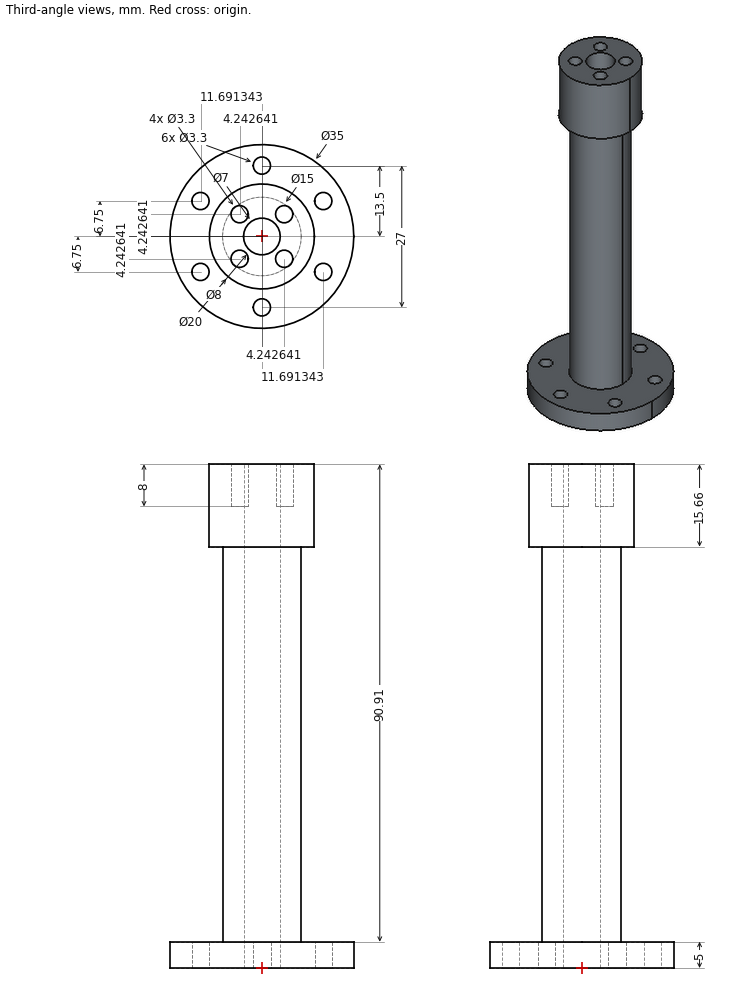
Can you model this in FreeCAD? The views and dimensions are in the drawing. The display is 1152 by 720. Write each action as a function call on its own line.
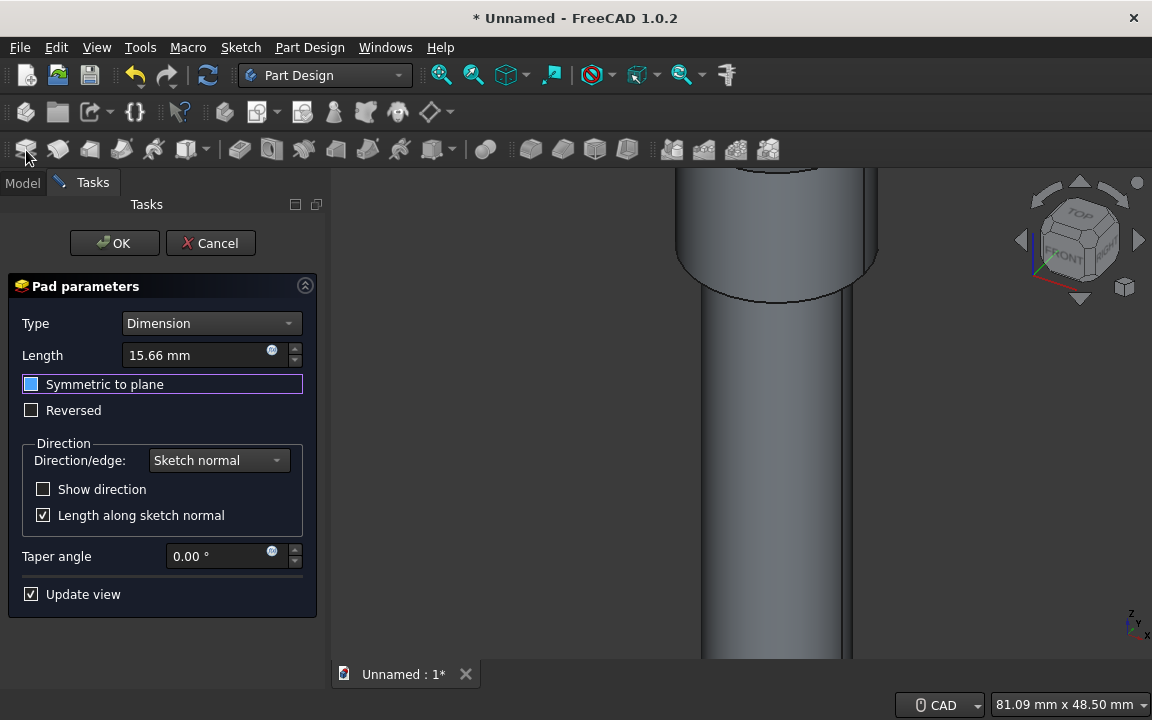
click(30, 410)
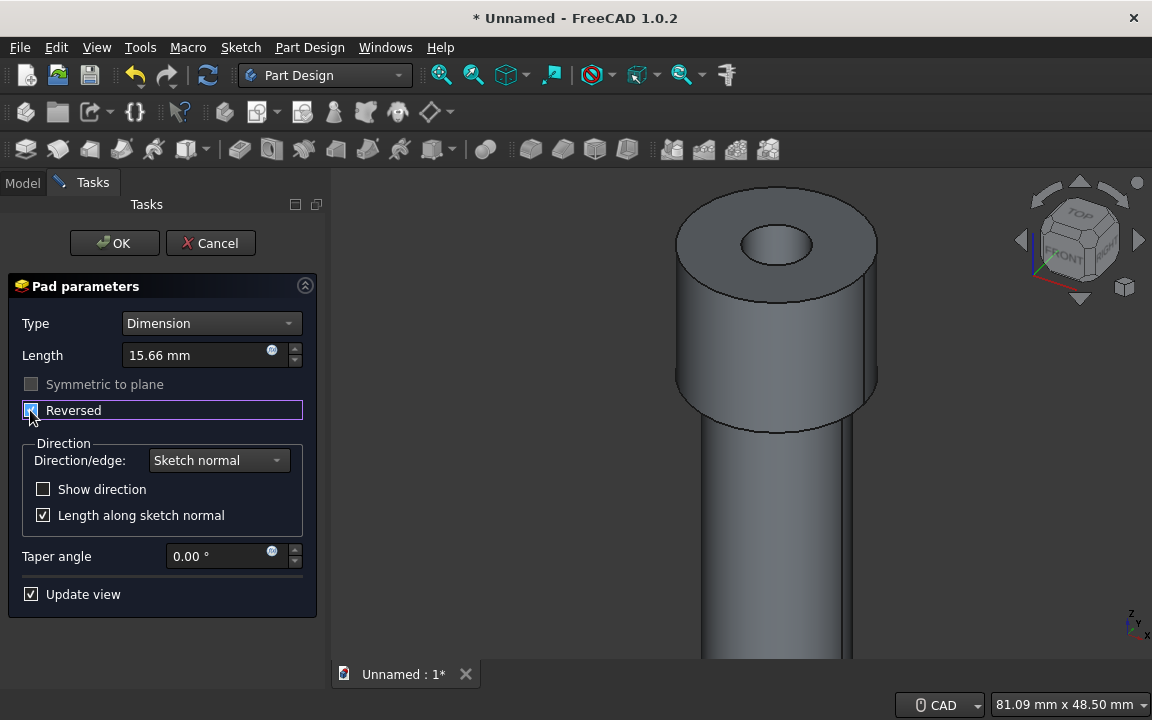
click(115, 243)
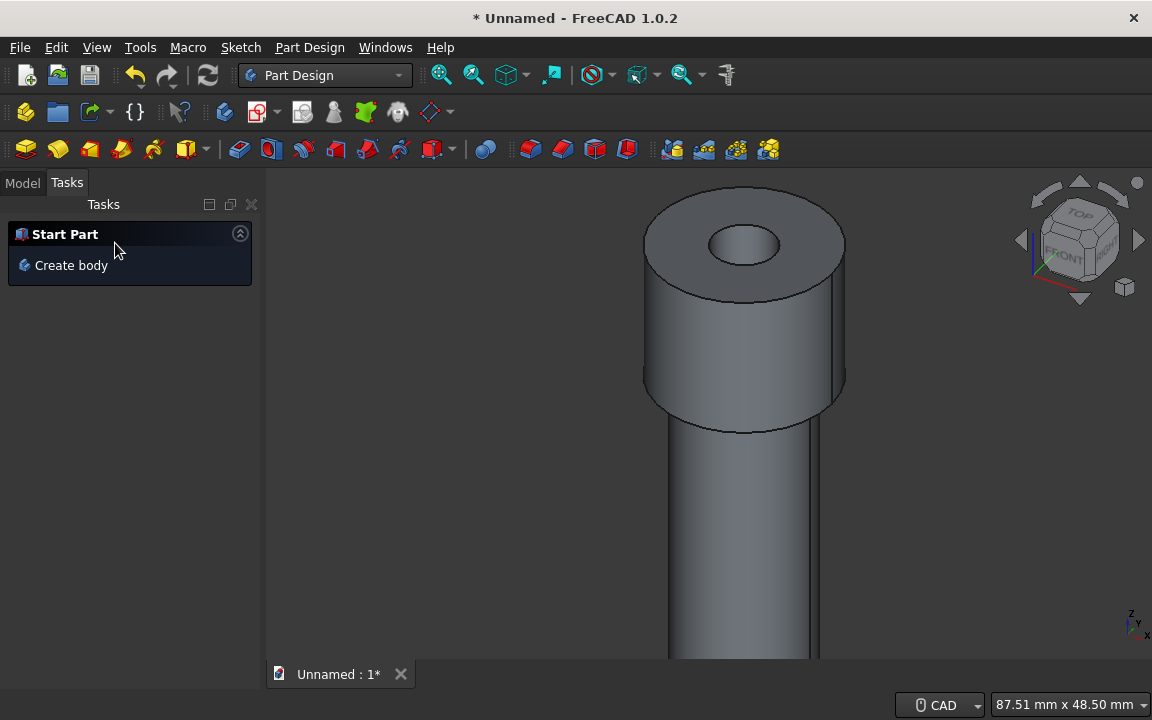
key(v)
key(f)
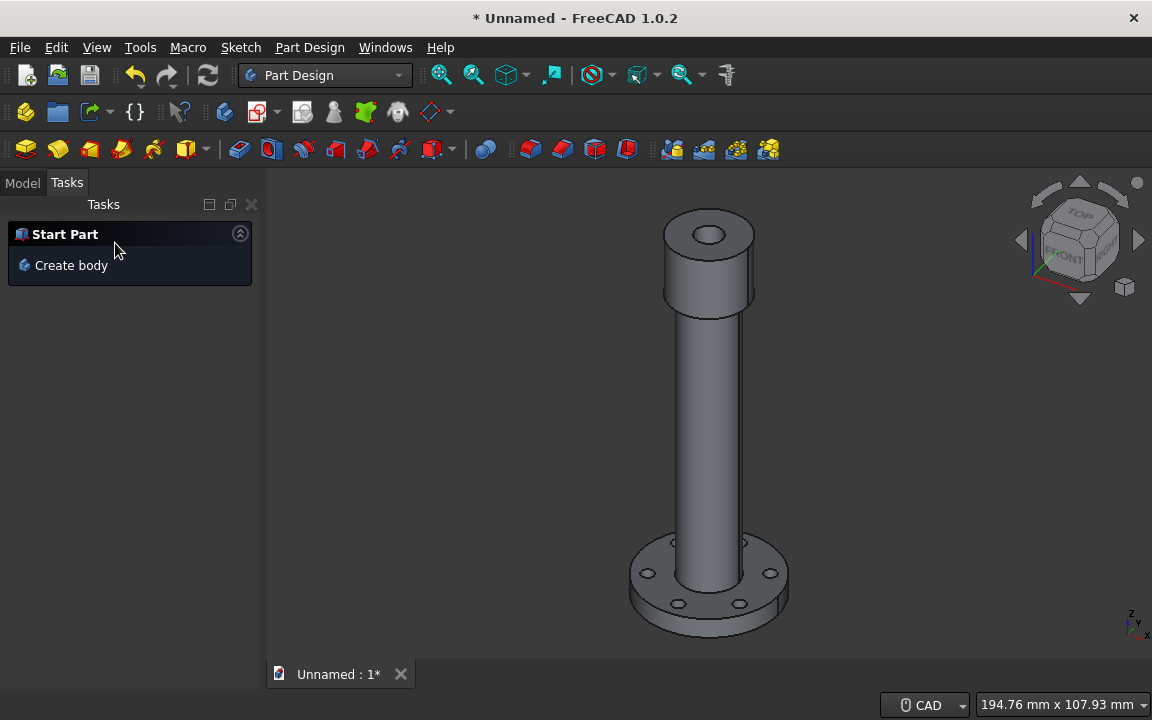
click(680, 233)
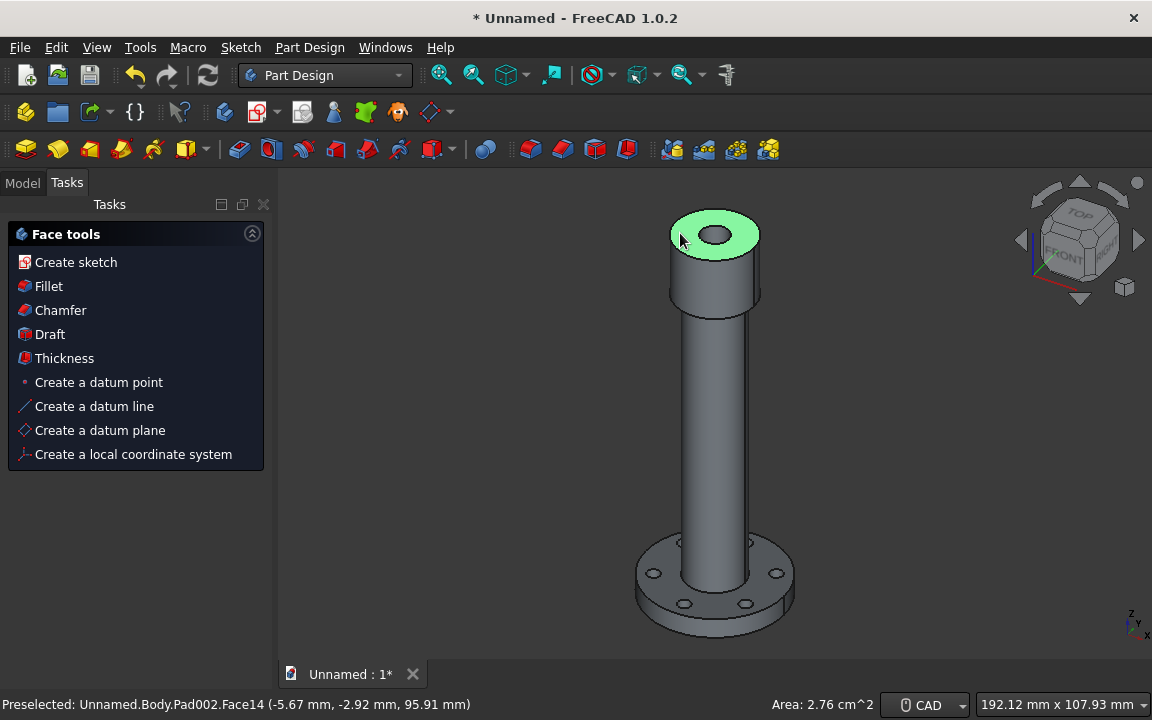
click(258, 112)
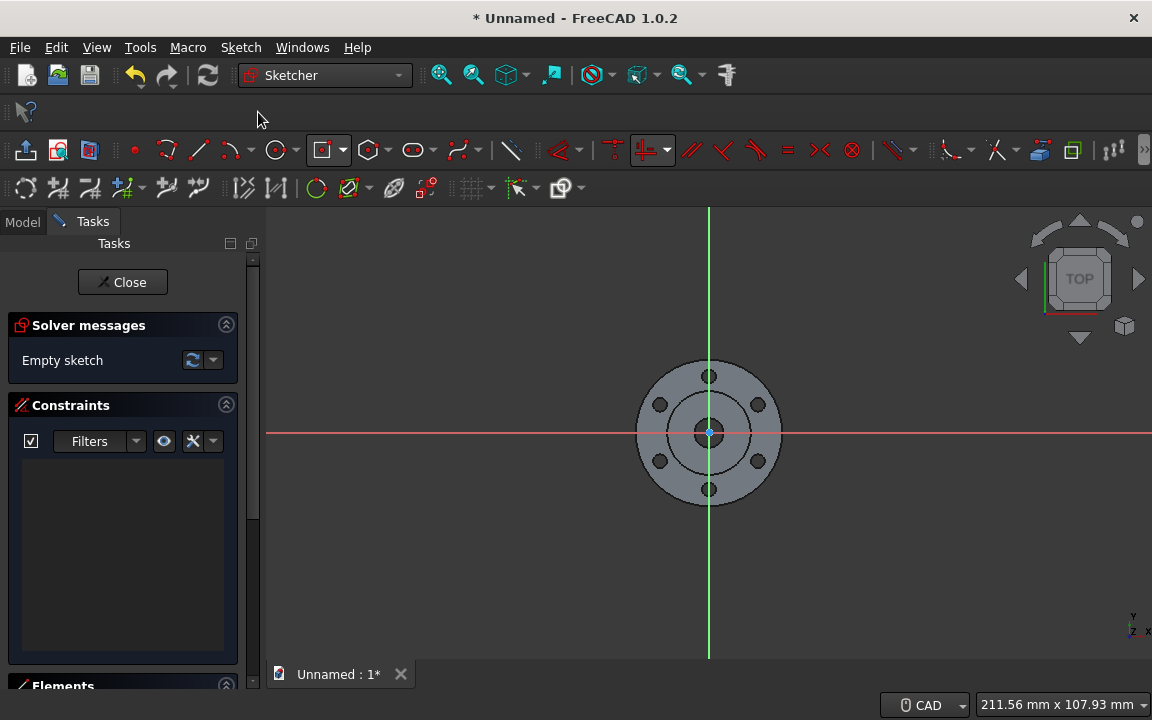
scroll(723, 433, up, 9)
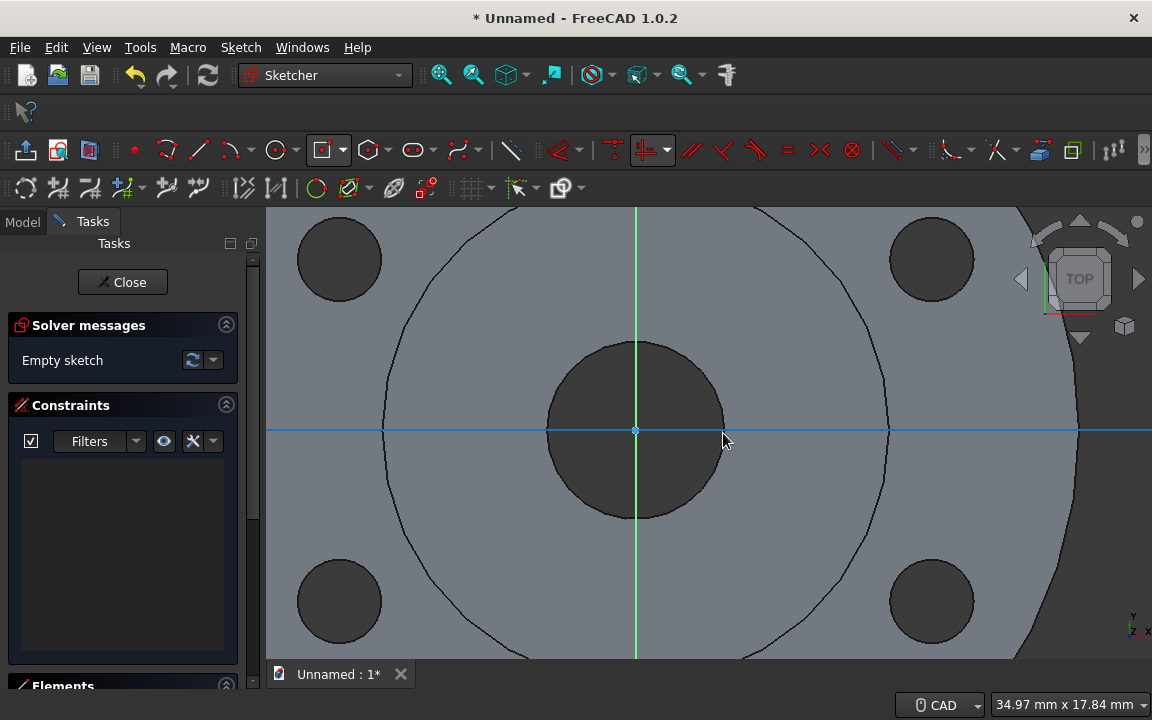
click(276, 150)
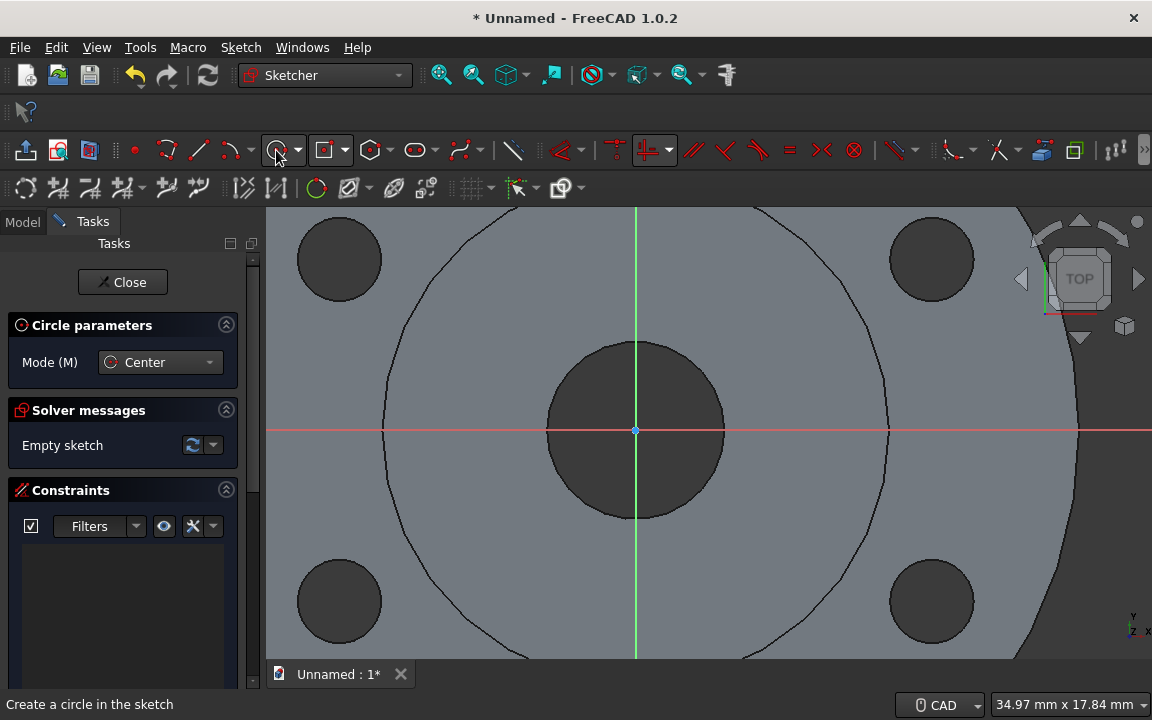
click(528, 323)
click(558, 293)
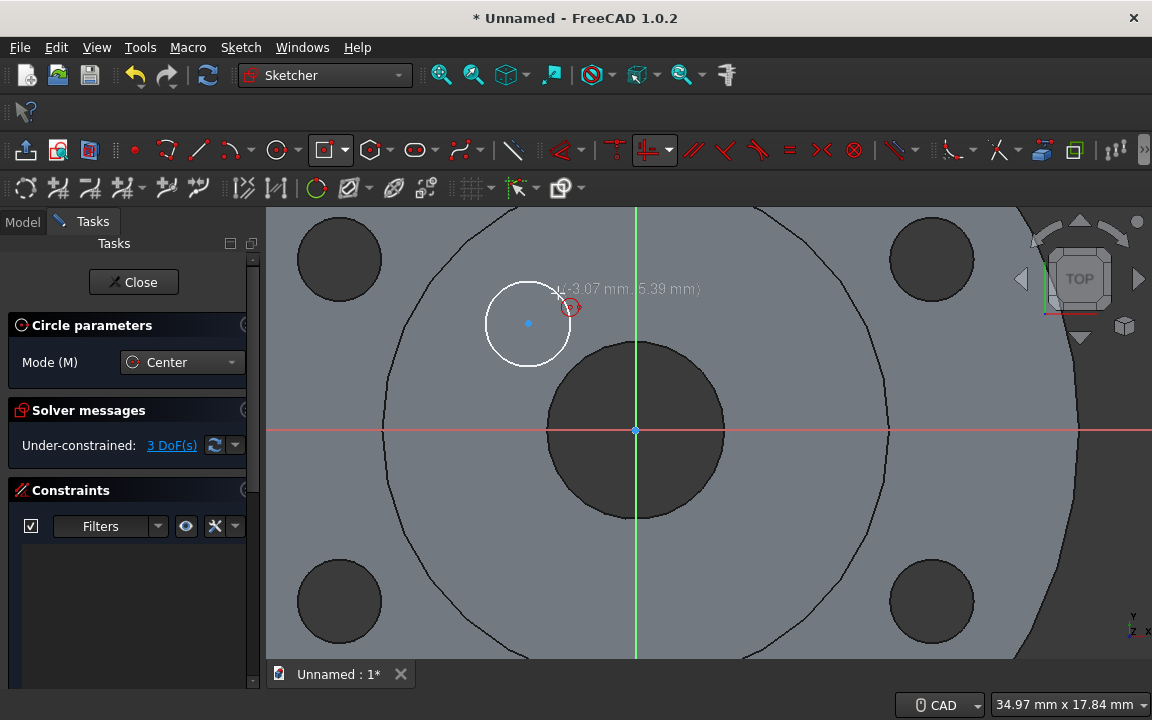
click(528, 538)
click(558, 508)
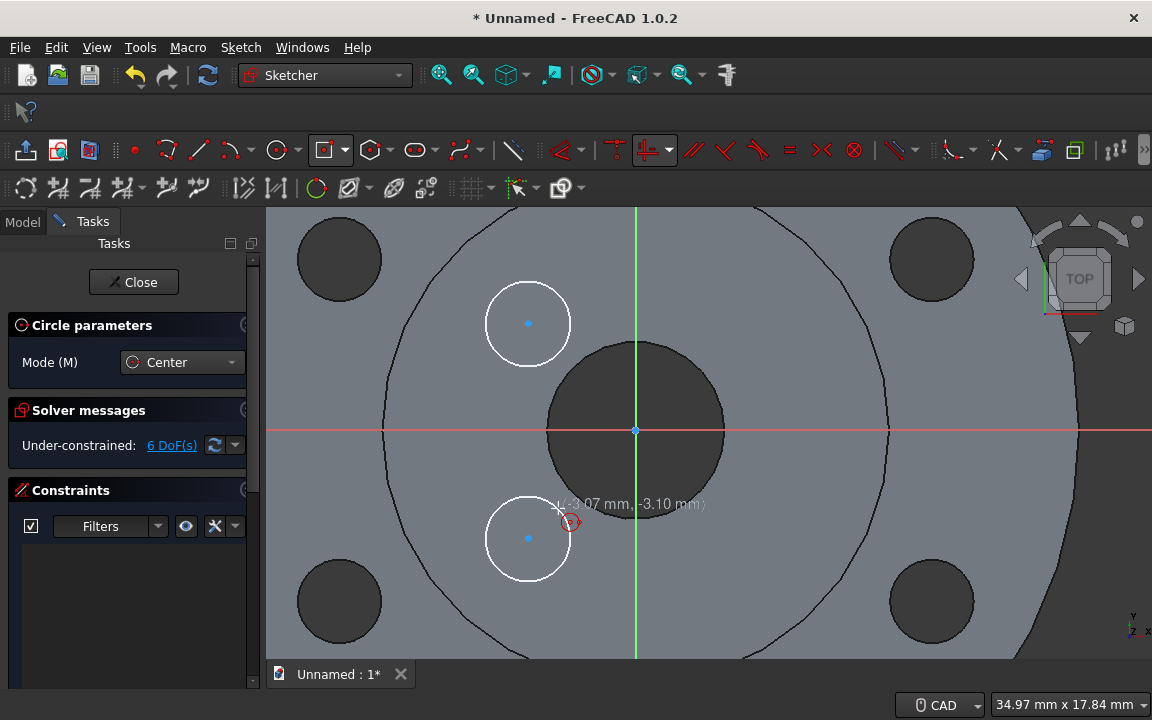
click(743, 538)
click(773, 508)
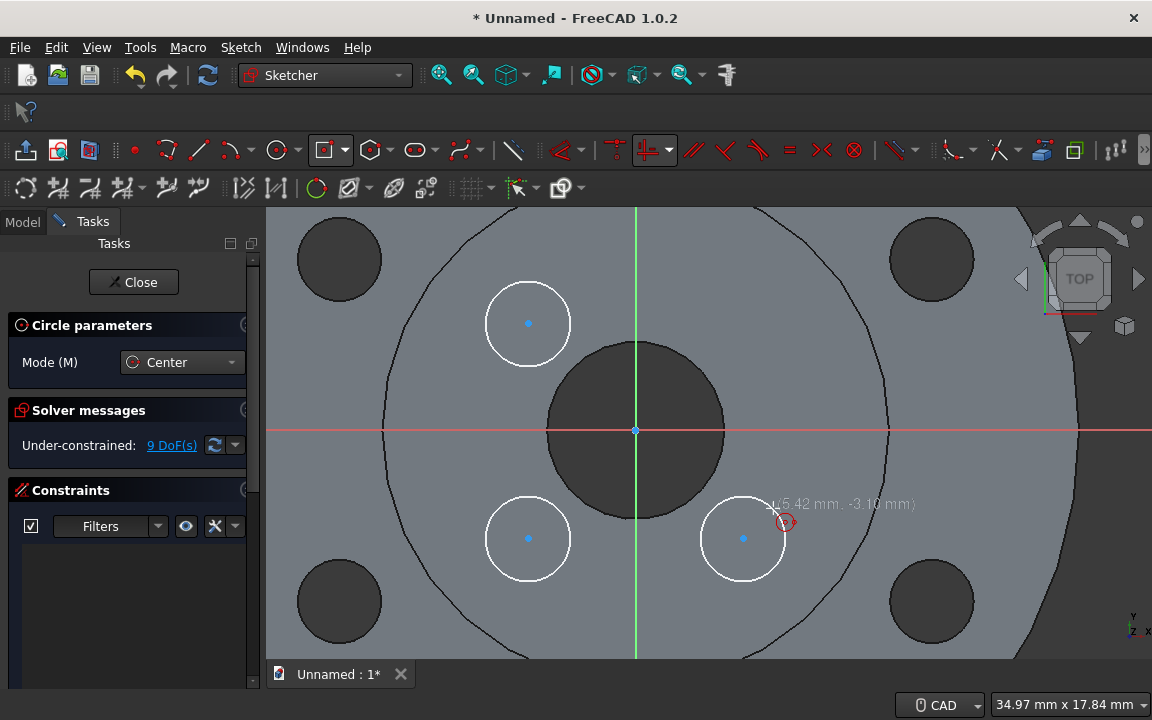
click(743, 323)
click(773, 293)
key(Escape)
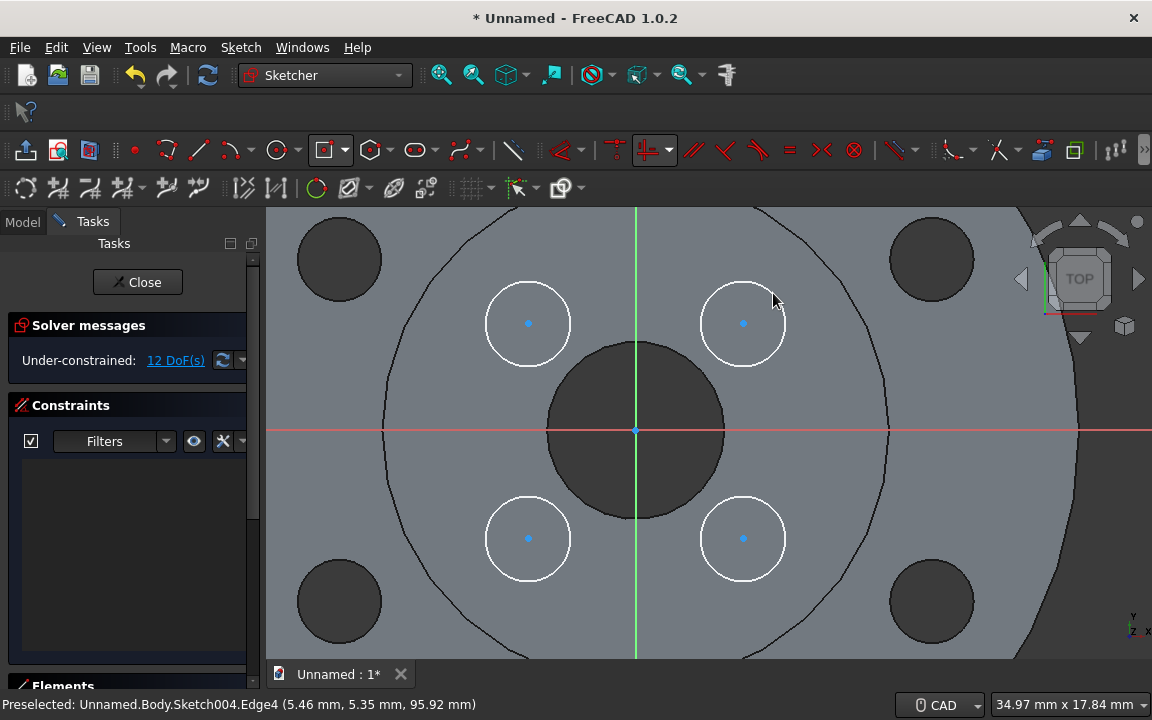
click(558, 294)